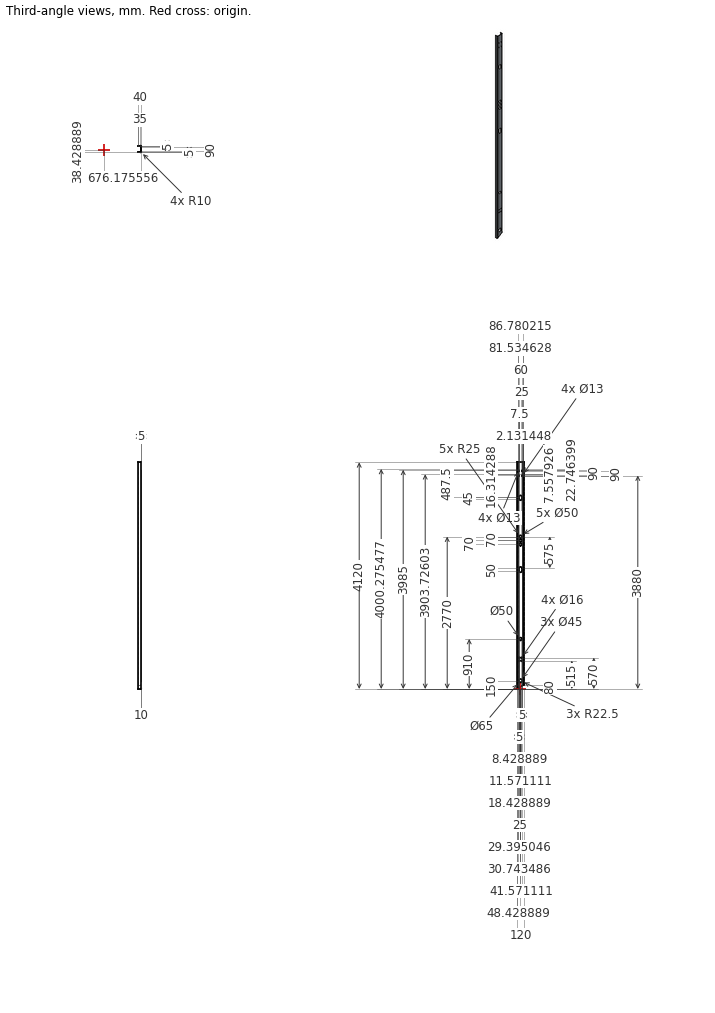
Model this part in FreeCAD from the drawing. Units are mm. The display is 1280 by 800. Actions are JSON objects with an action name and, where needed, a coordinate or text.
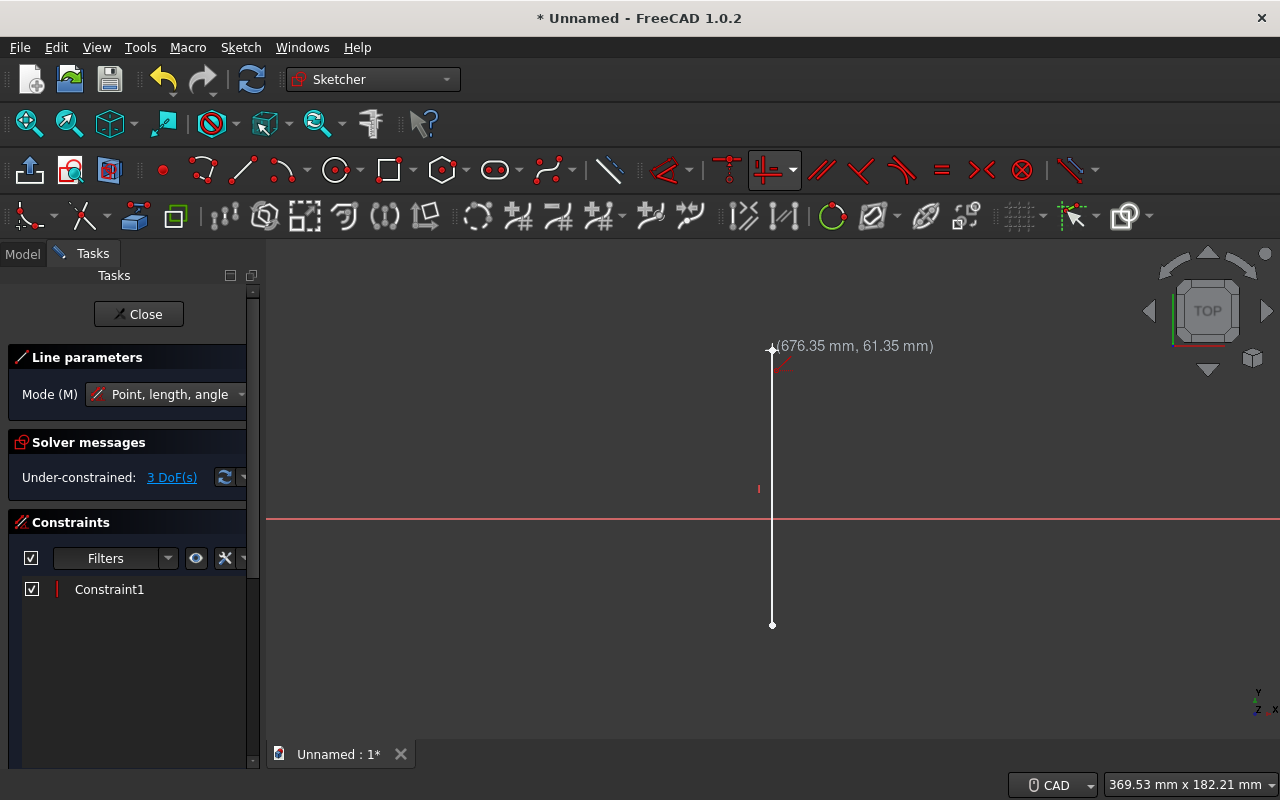
{"action": "key", "text": "g m"}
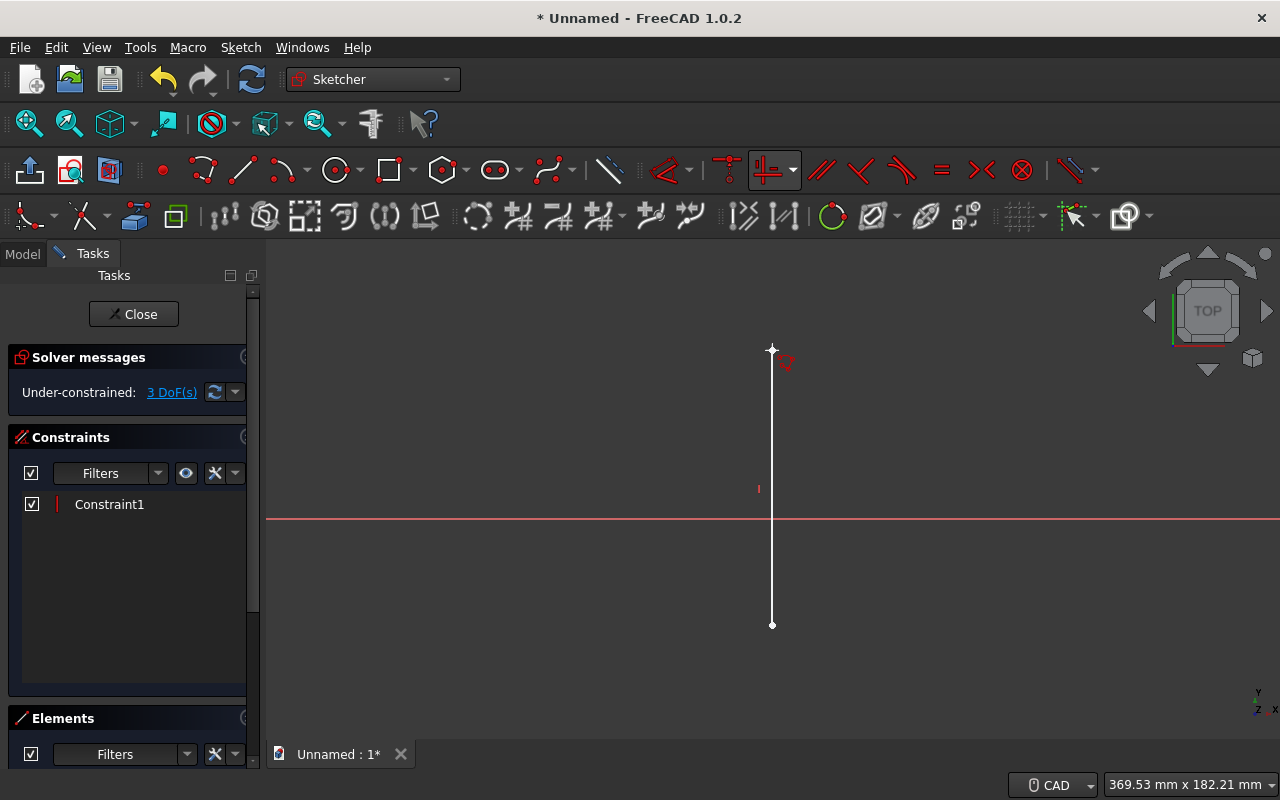
{"action": "left_click", "coordinate": [744, 323]}
{"action": "left_click", "coordinate": [634, 323]}
{"action": "left_click", "coordinate": [634, 337]}
{"action": "left_click", "coordinate": [730, 337]}
{"action": "right_click", "coordinate": [730, 337]}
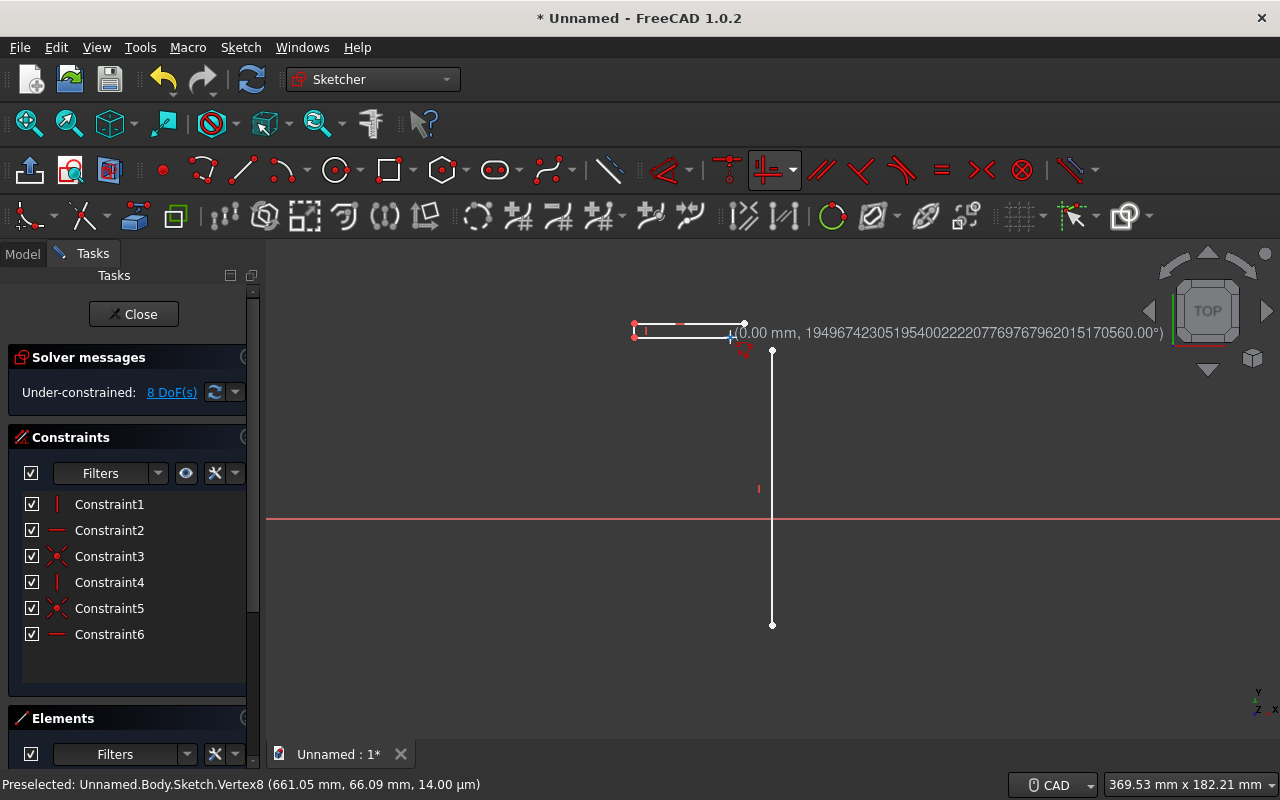
{"action": "key", "text": "g l"}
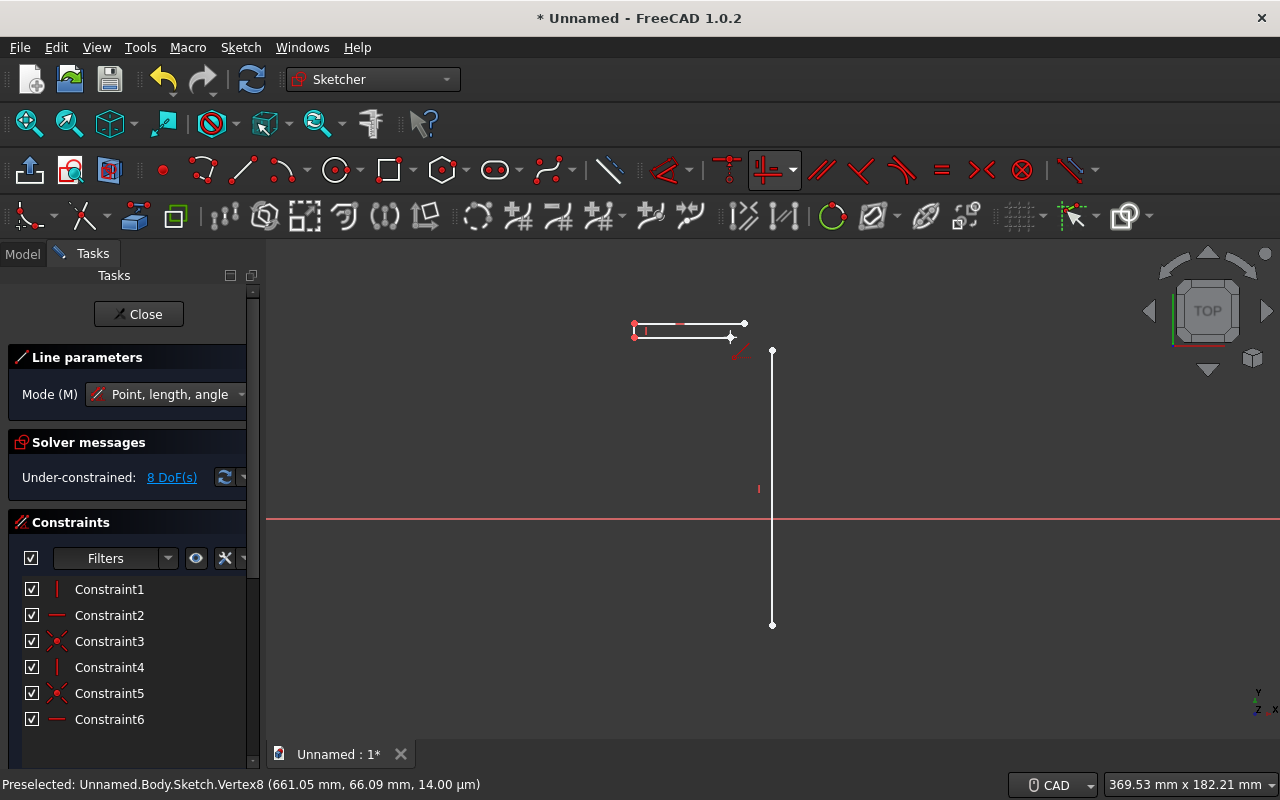
{"action": "left_click", "coordinate": [758, 364]}
{"action": "left_click", "coordinate": [758, 611]}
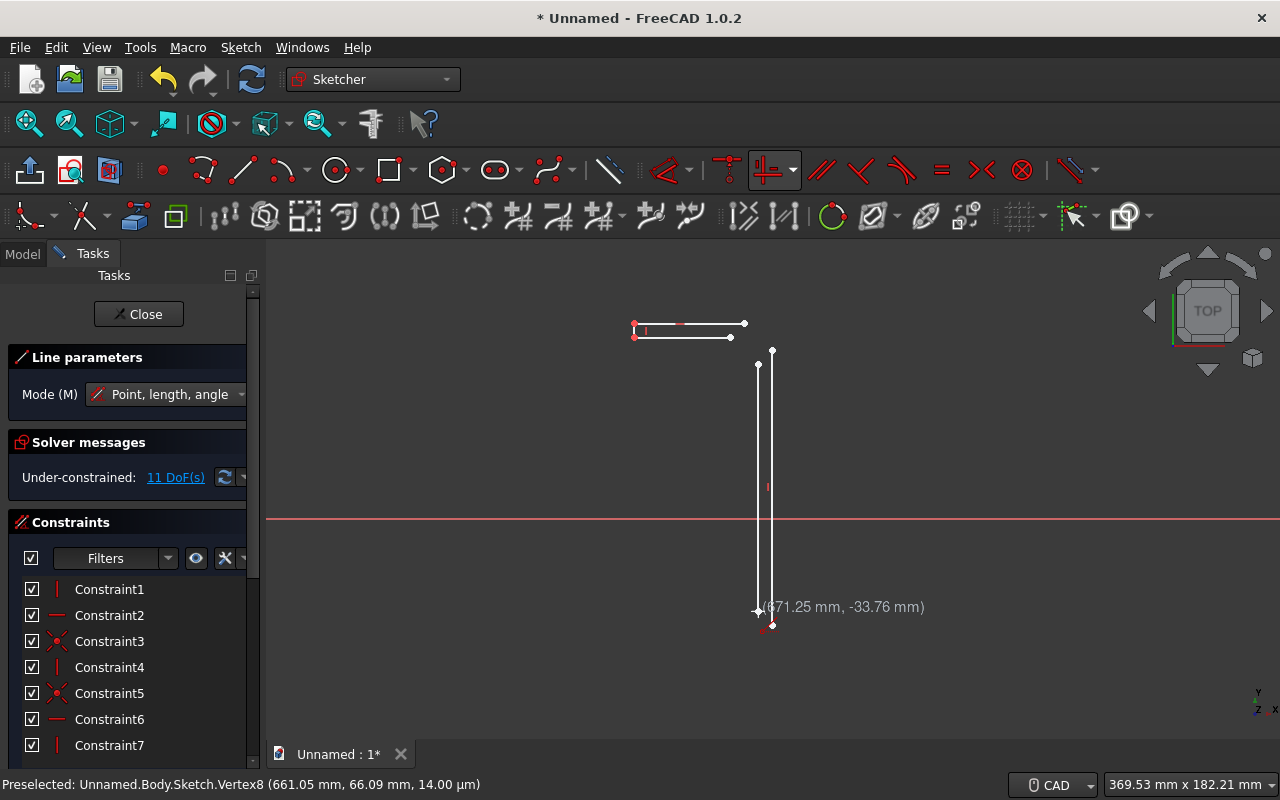
{"action": "left_click", "coordinate": [204, 170]}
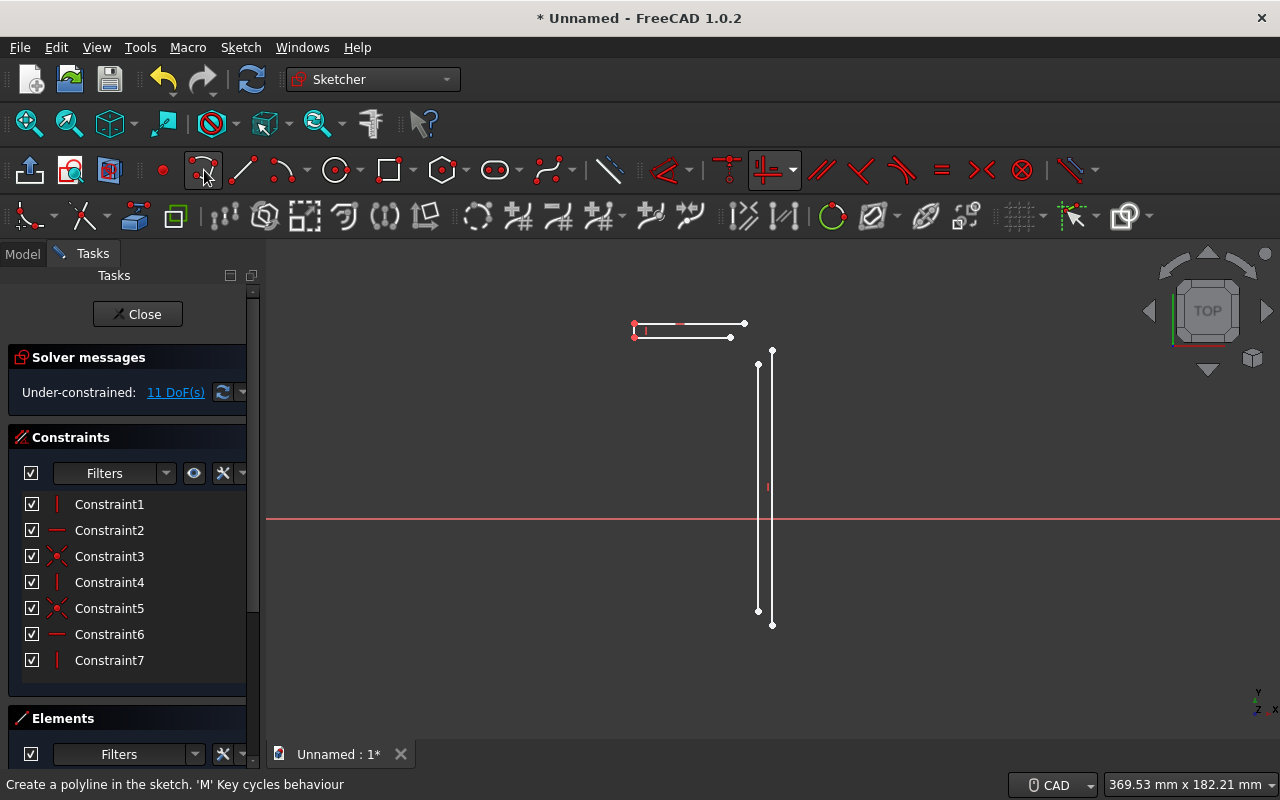
{"action": "left_click", "coordinate": [730, 639]}
{"action": "left_click", "coordinate": [634, 639]}
{"action": "left_click", "coordinate": [634, 652]}
{"action": "left_click", "coordinate": [744, 652]}
{"action": "right_click", "coordinate": [744, 652]}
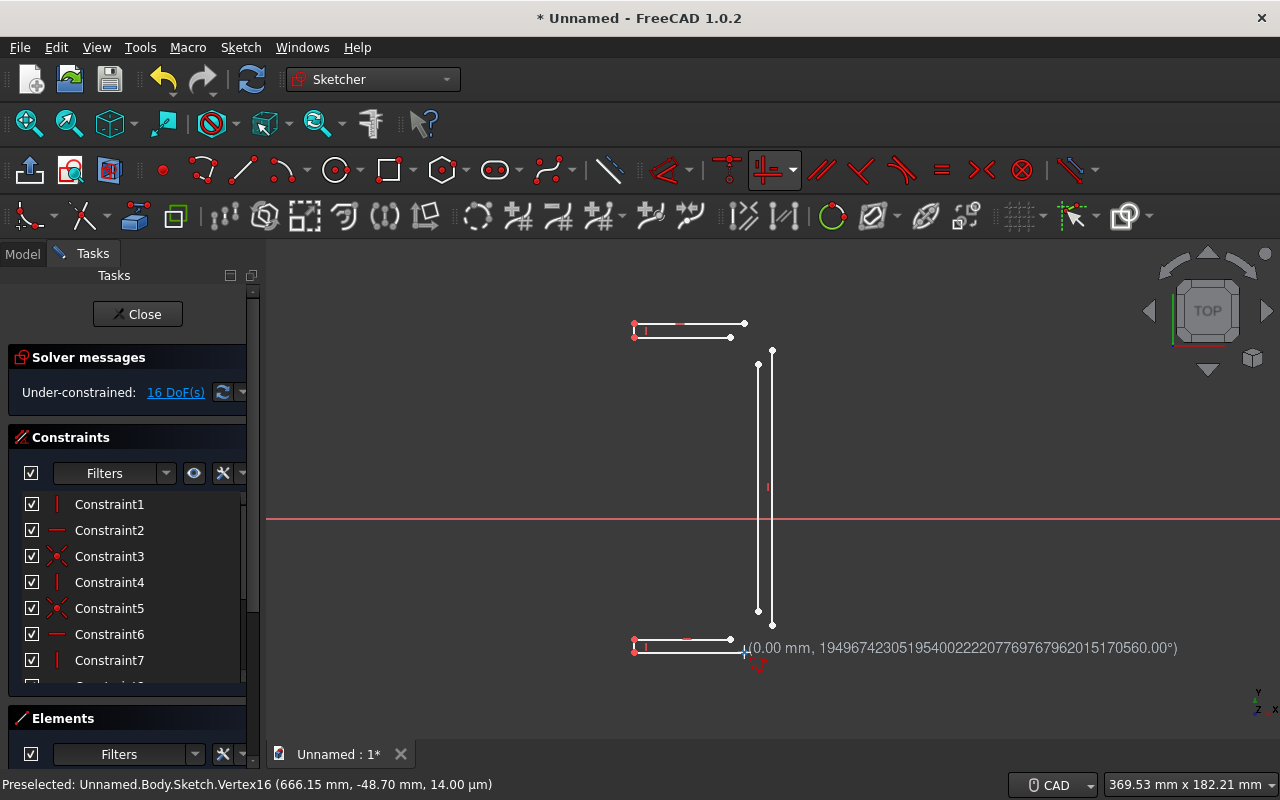
{"action": "key", "text": "g 3 a"}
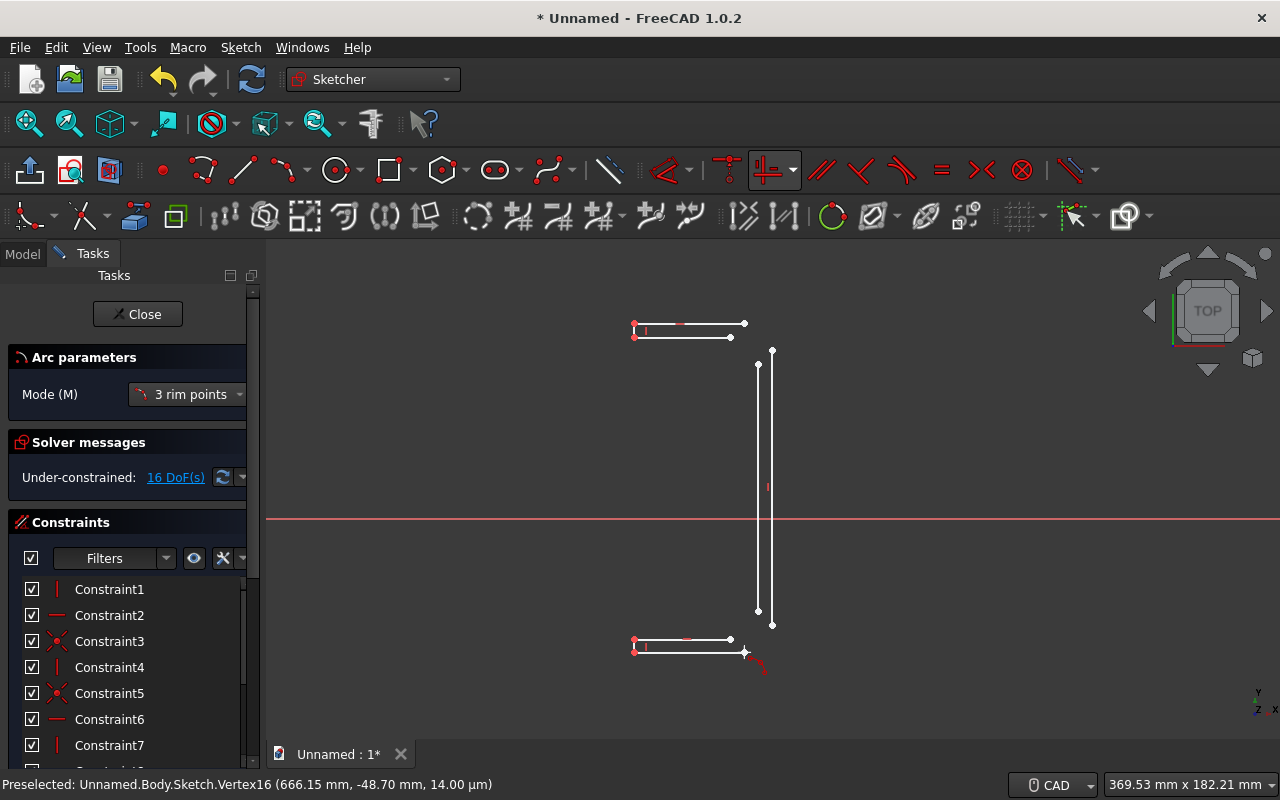
{"action": "left_click", "coordinate": [772, 351]}
{"action": "left_click", "coordinate": [744, 324]}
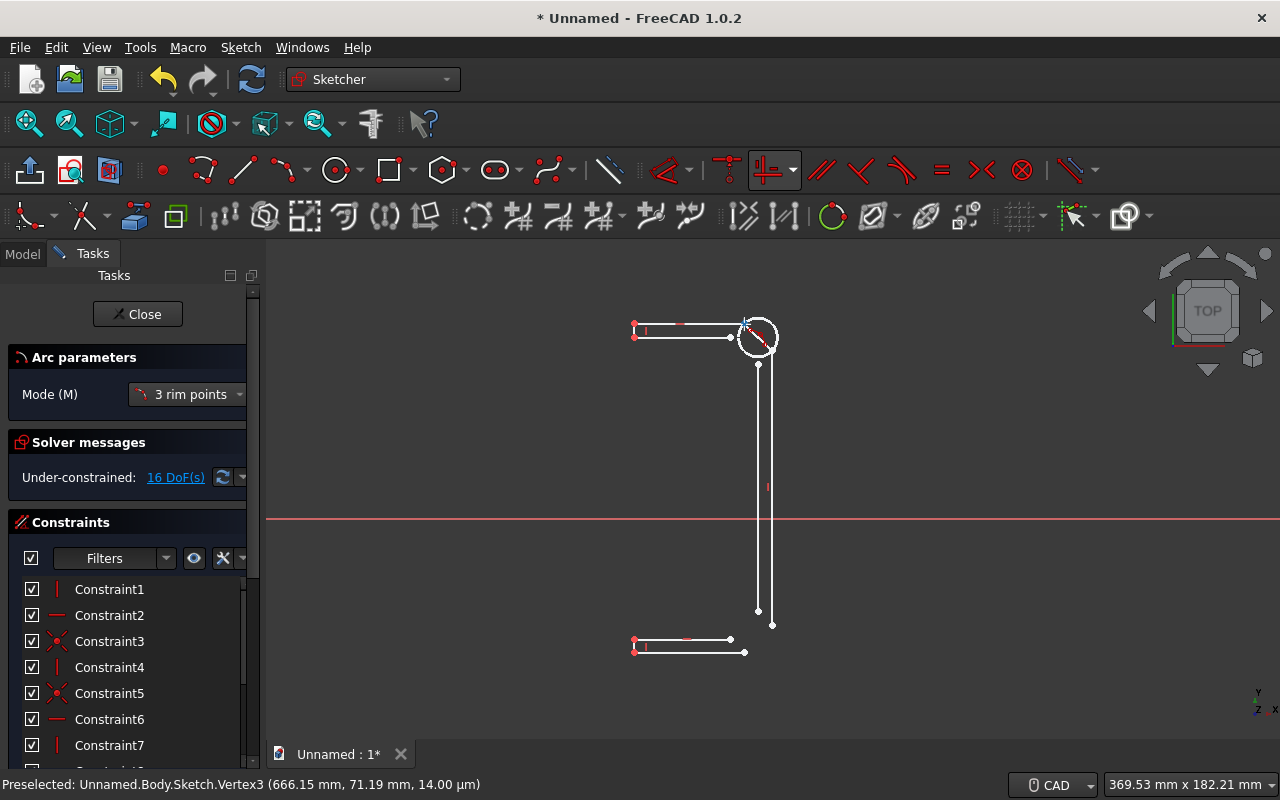
{"action": "scroll", "coordinate": [763, 331], "scroll_direction": "up", "scroll_amount": 4}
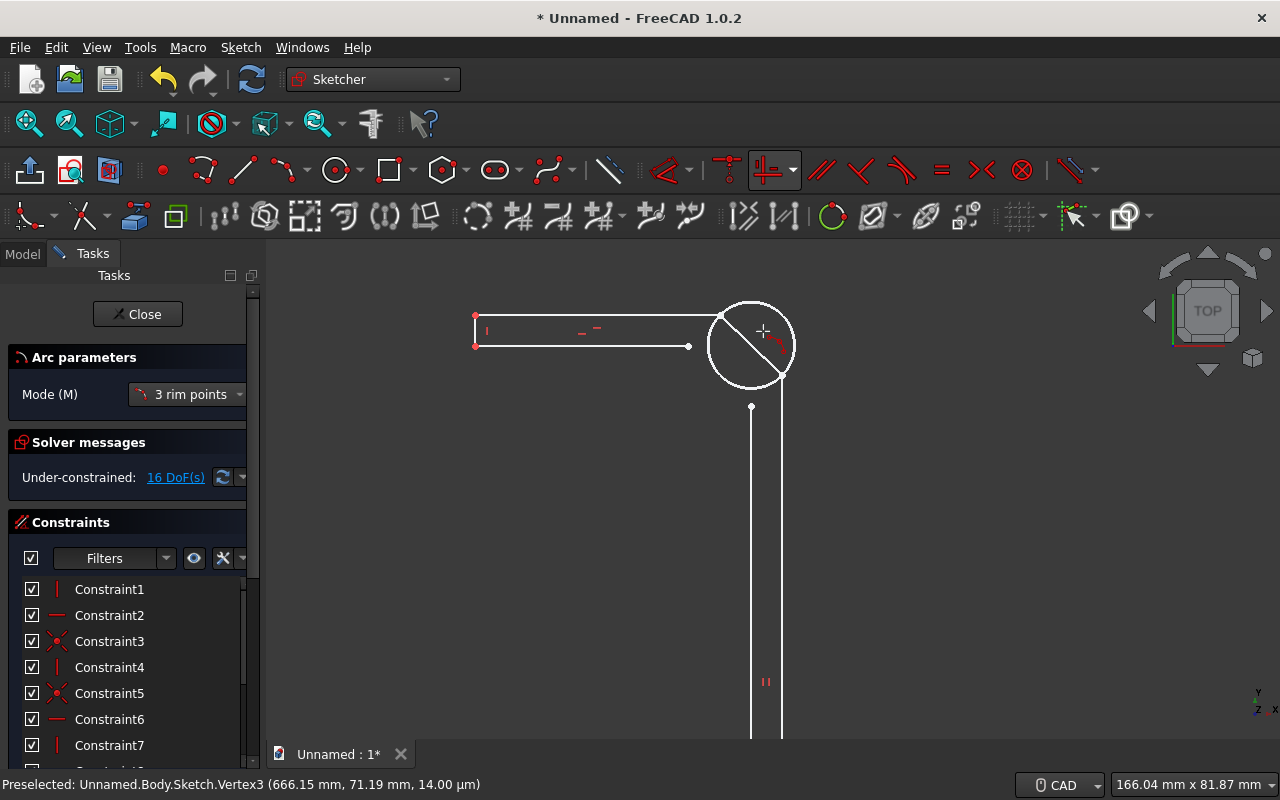
{"action": "left_click", "coordinate": [763, 331]}